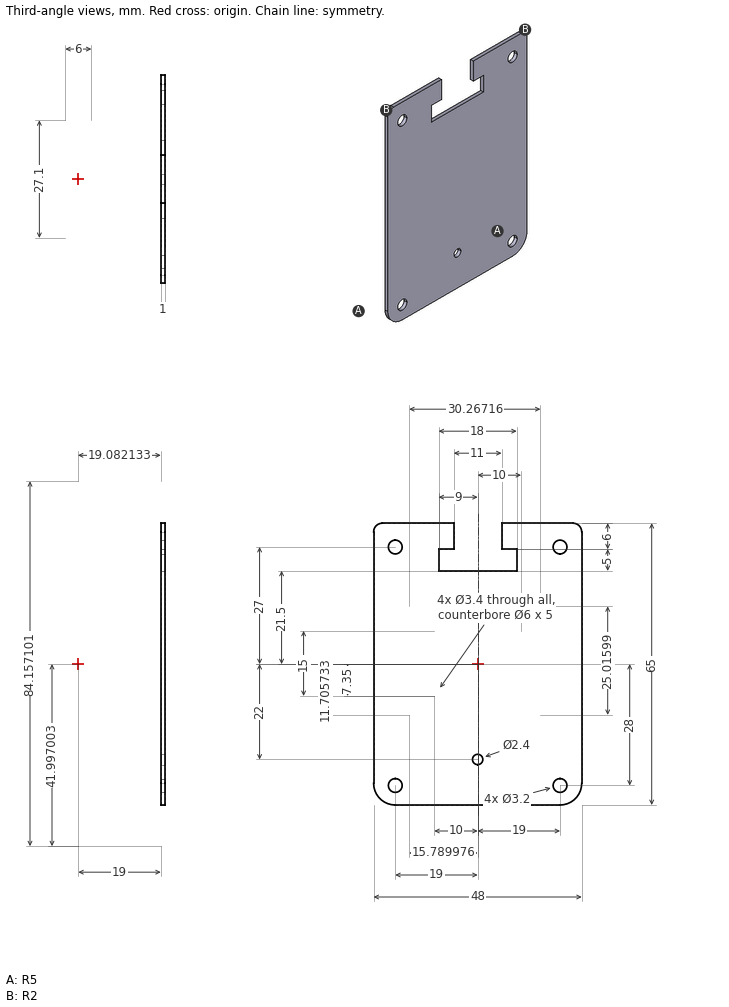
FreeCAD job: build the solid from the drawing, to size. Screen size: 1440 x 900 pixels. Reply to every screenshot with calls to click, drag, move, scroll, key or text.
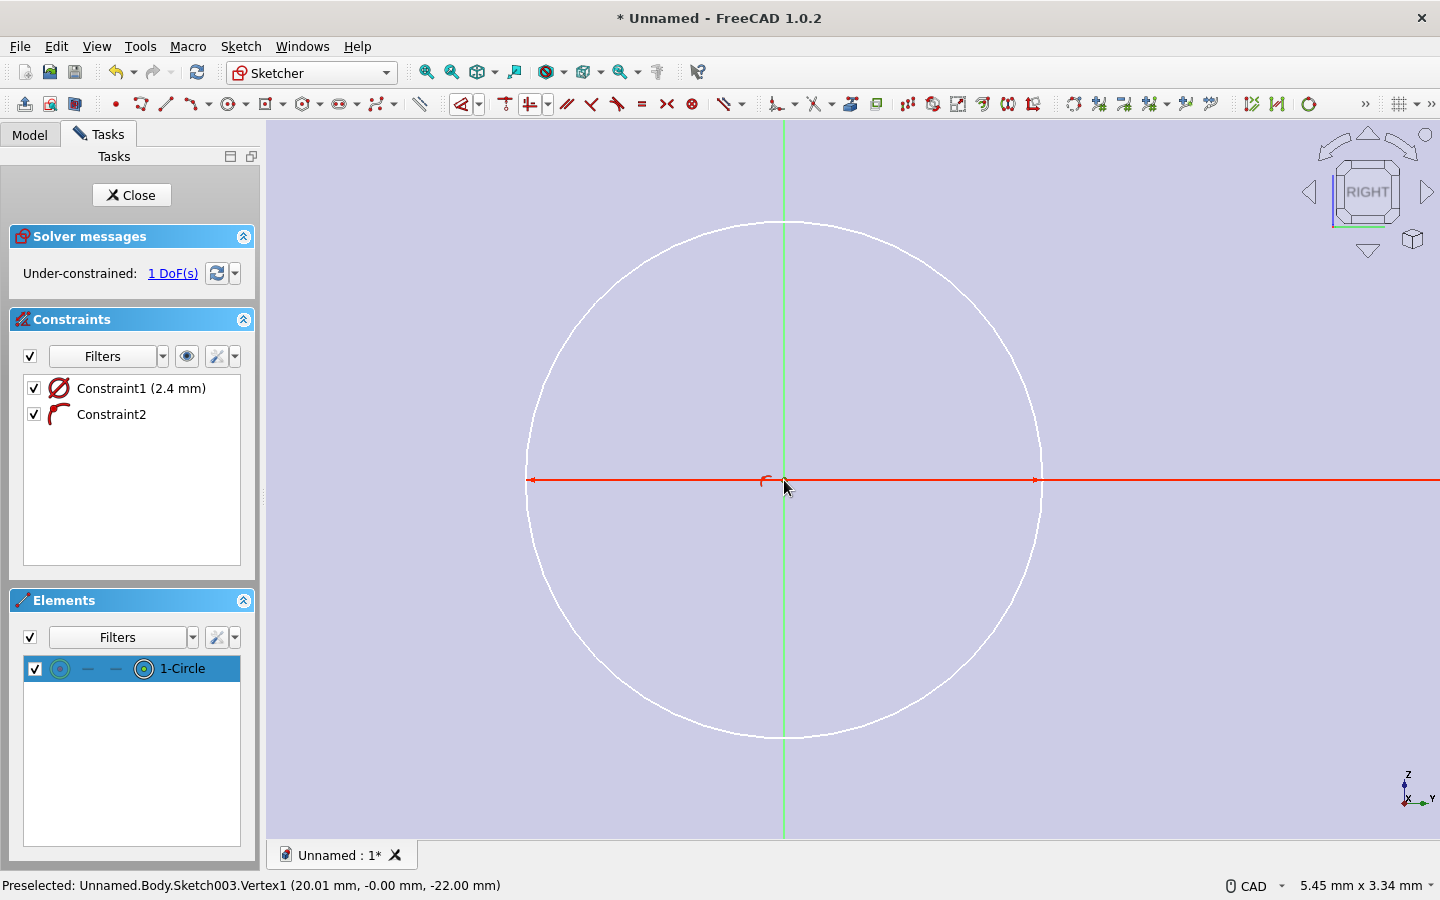
key(i)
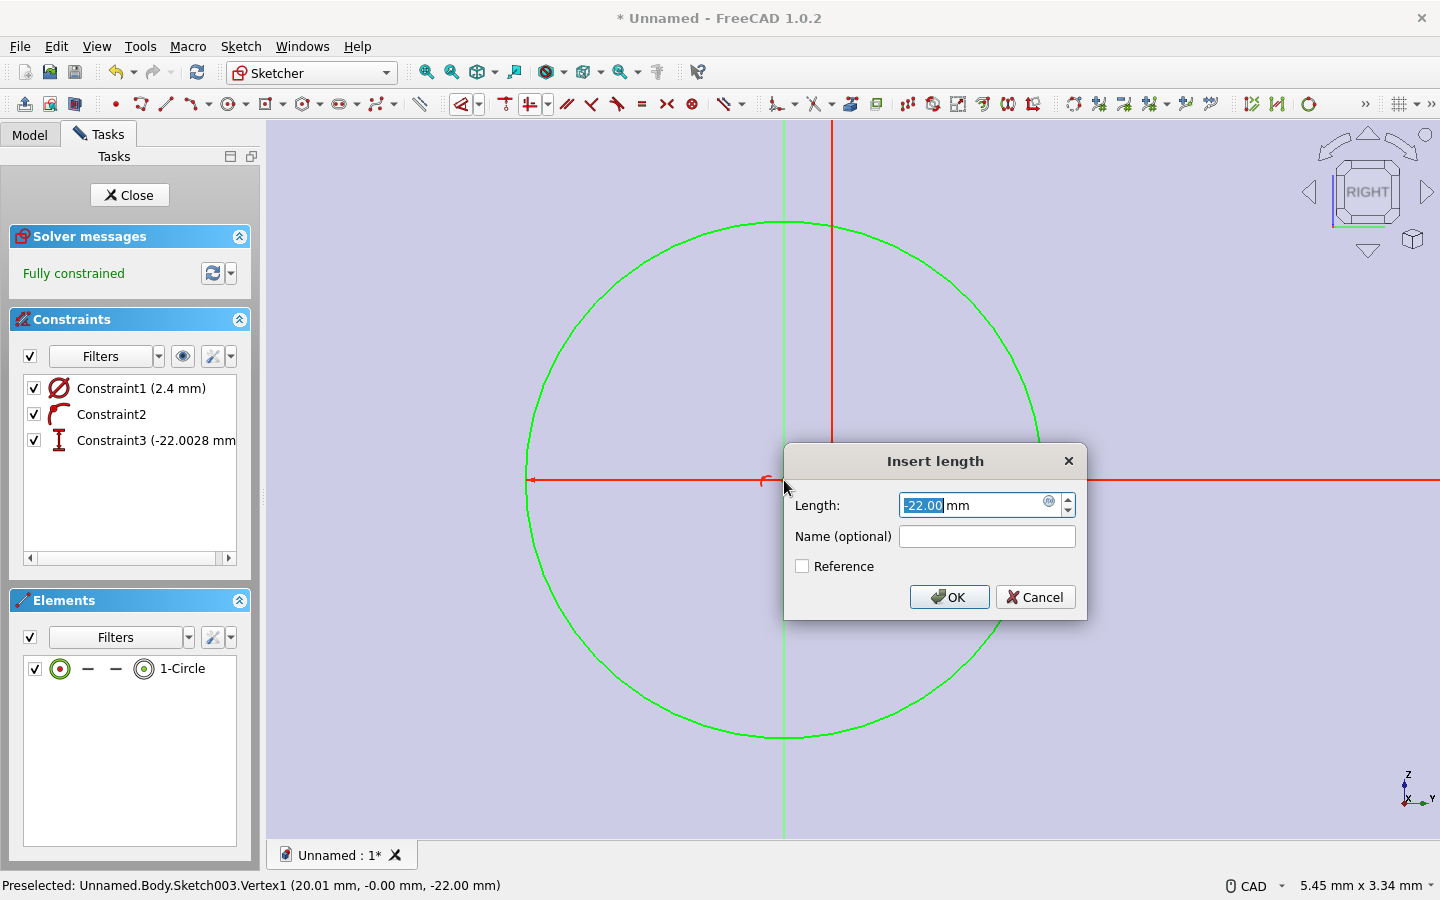
text(-22)
key(Return)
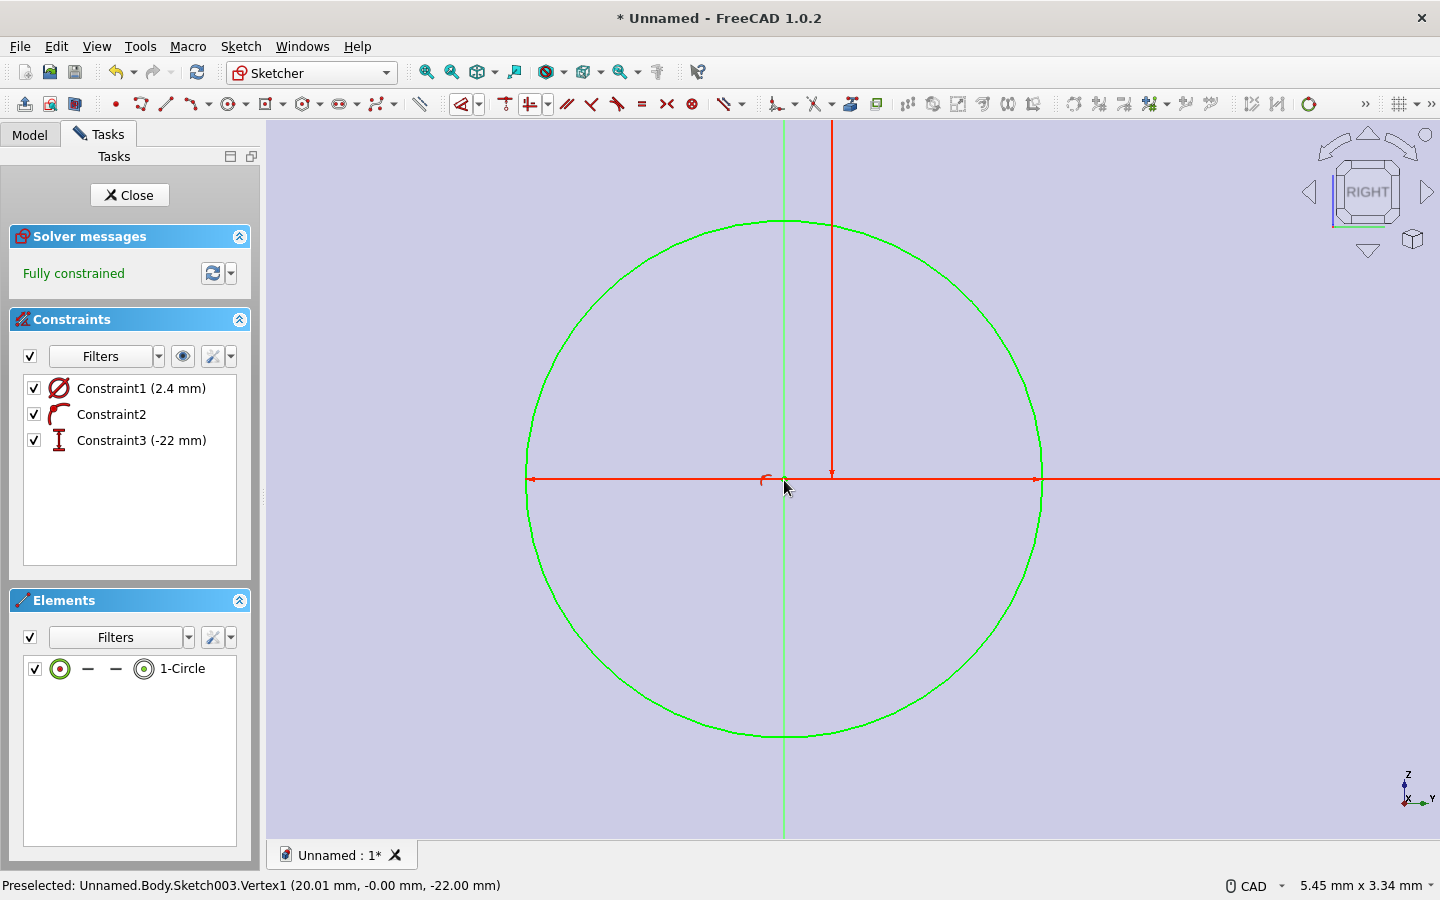
click(130, 195)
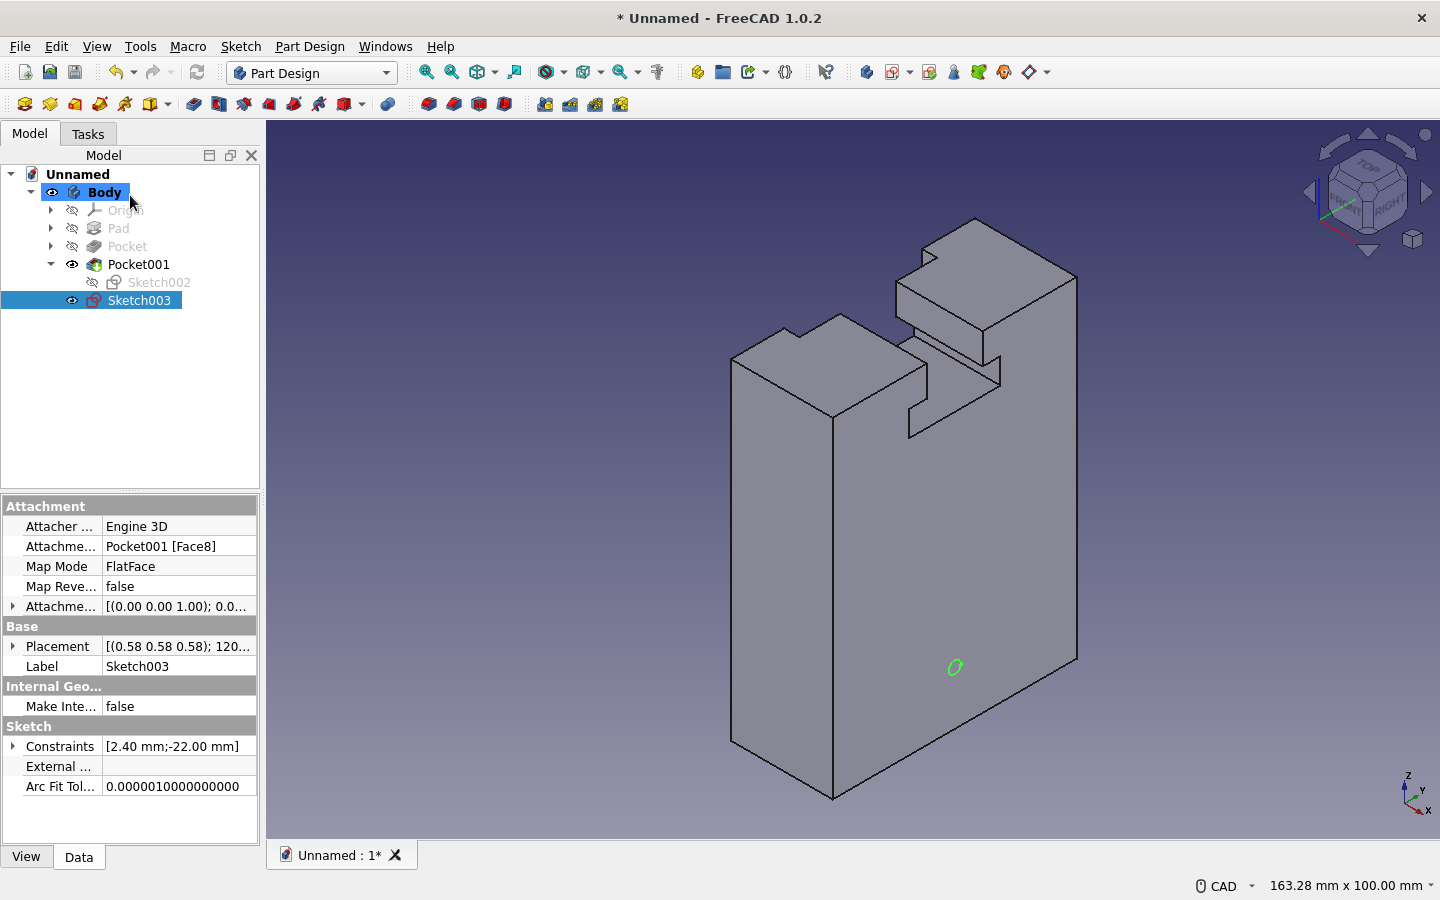
click(194, 104)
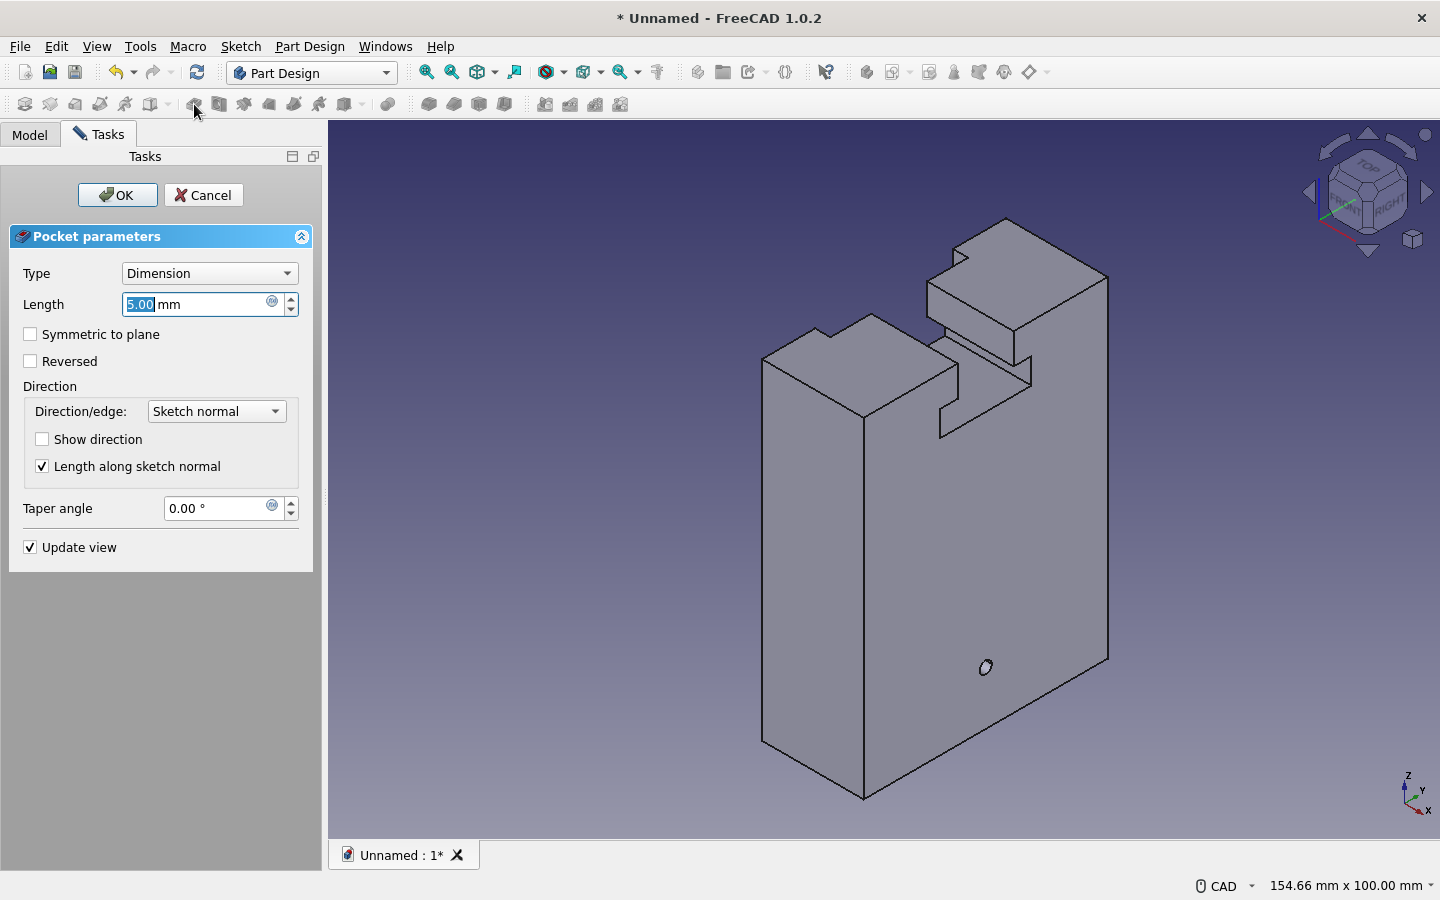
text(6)
key(Tab)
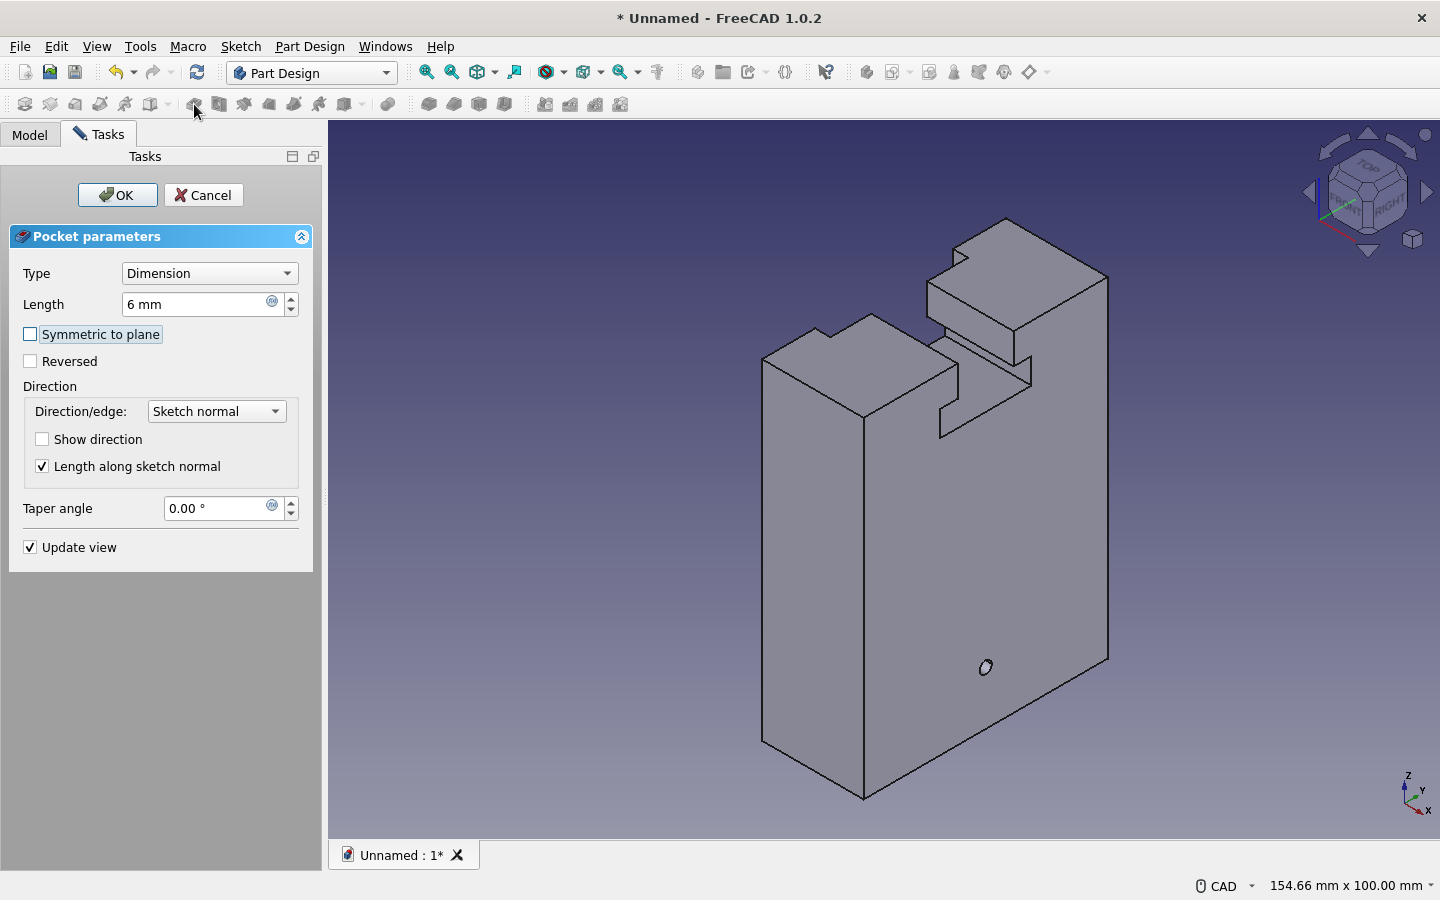
click(118, 195)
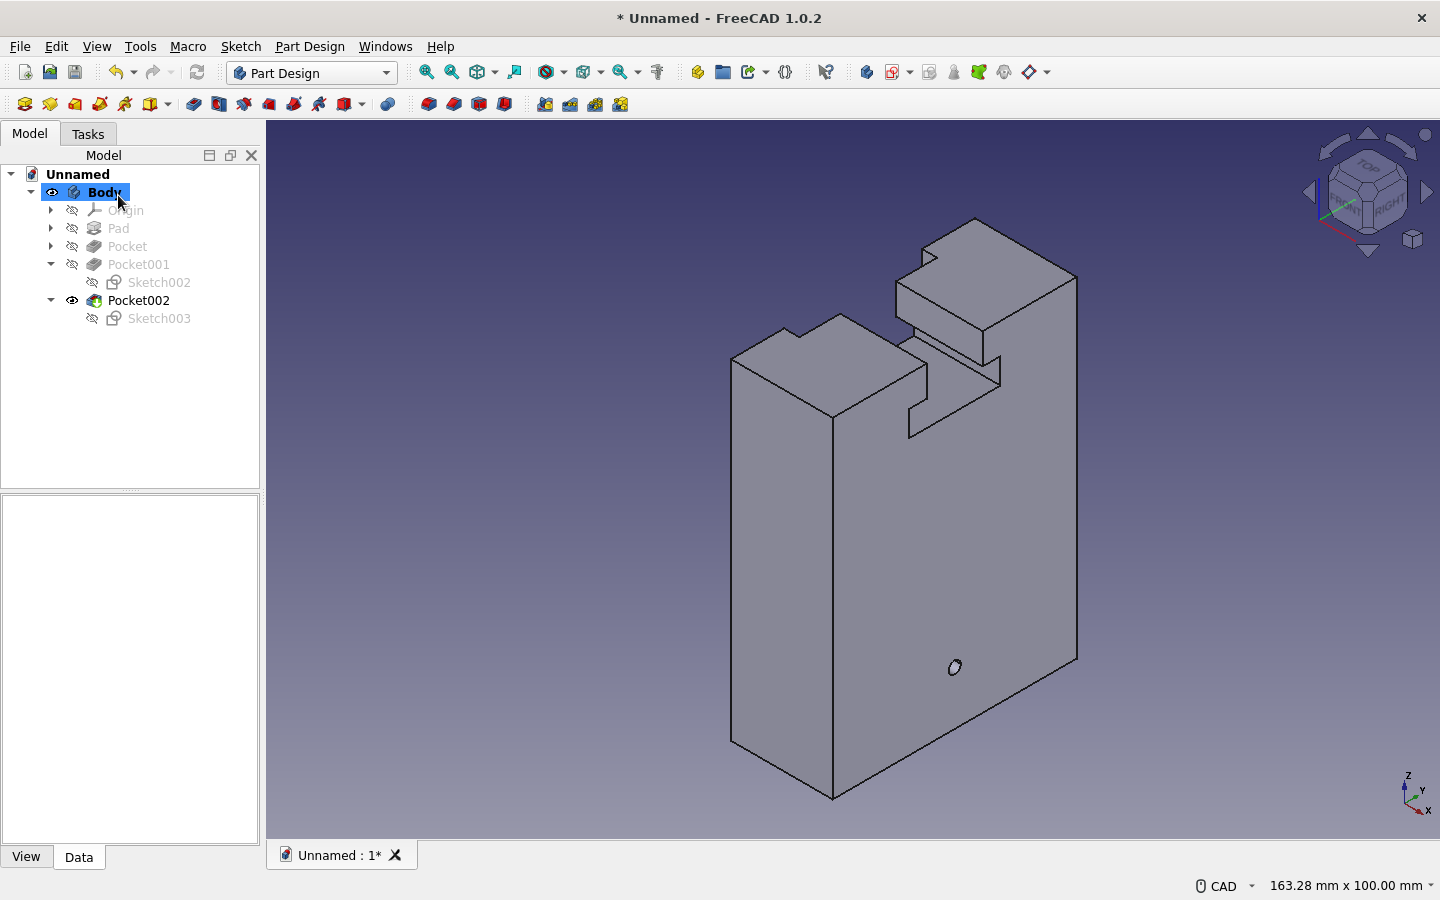
click(955, 537)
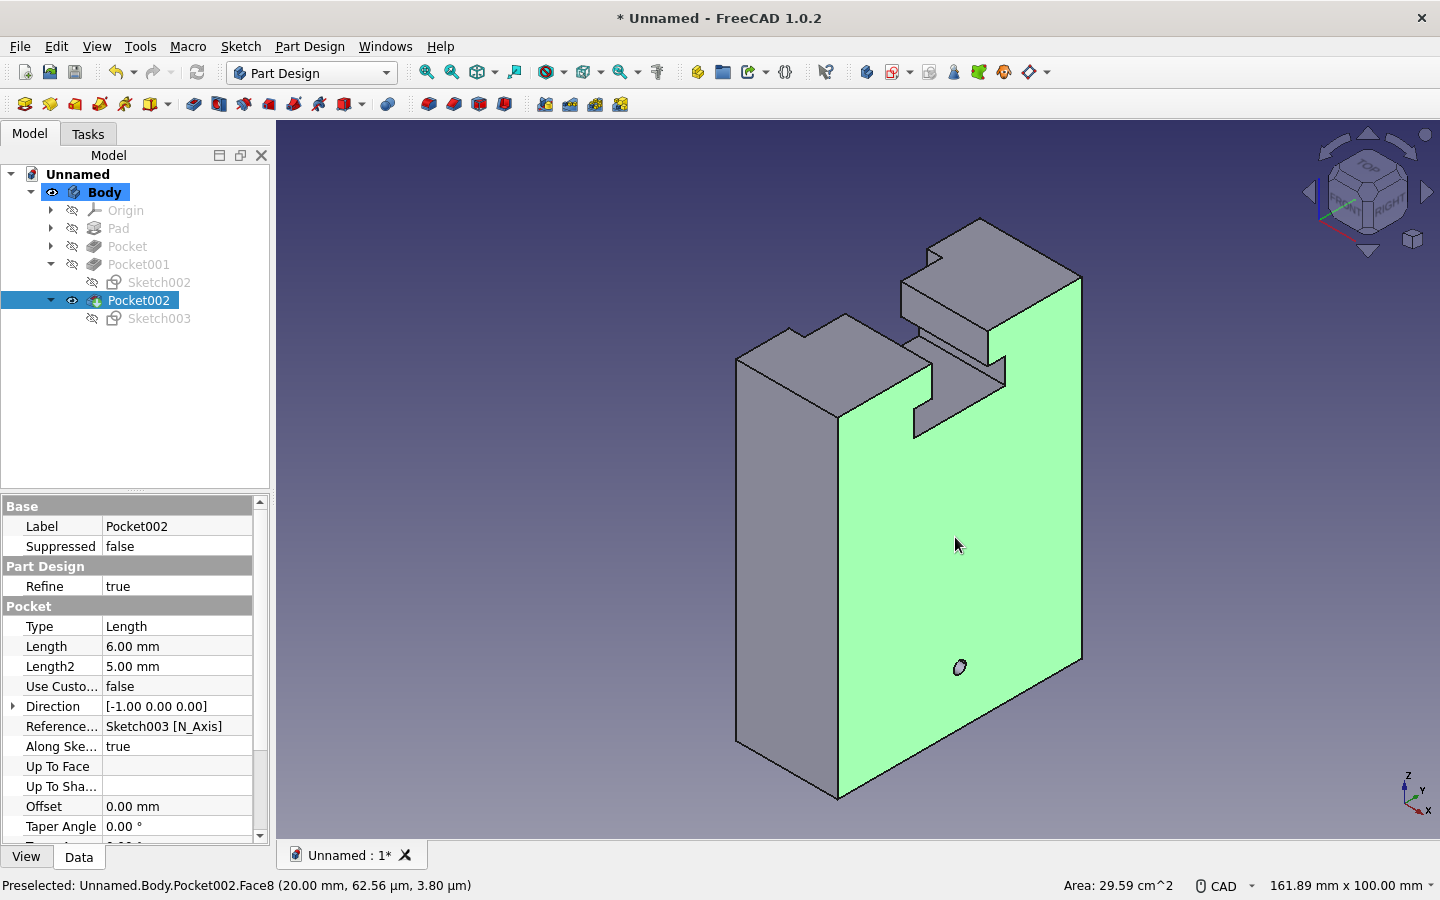
click(892, 72)